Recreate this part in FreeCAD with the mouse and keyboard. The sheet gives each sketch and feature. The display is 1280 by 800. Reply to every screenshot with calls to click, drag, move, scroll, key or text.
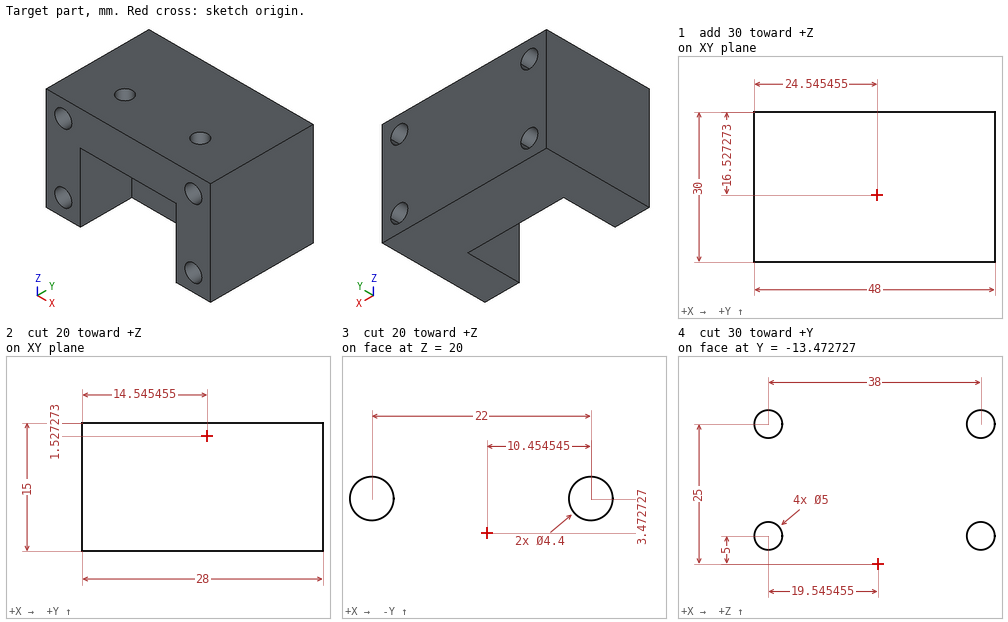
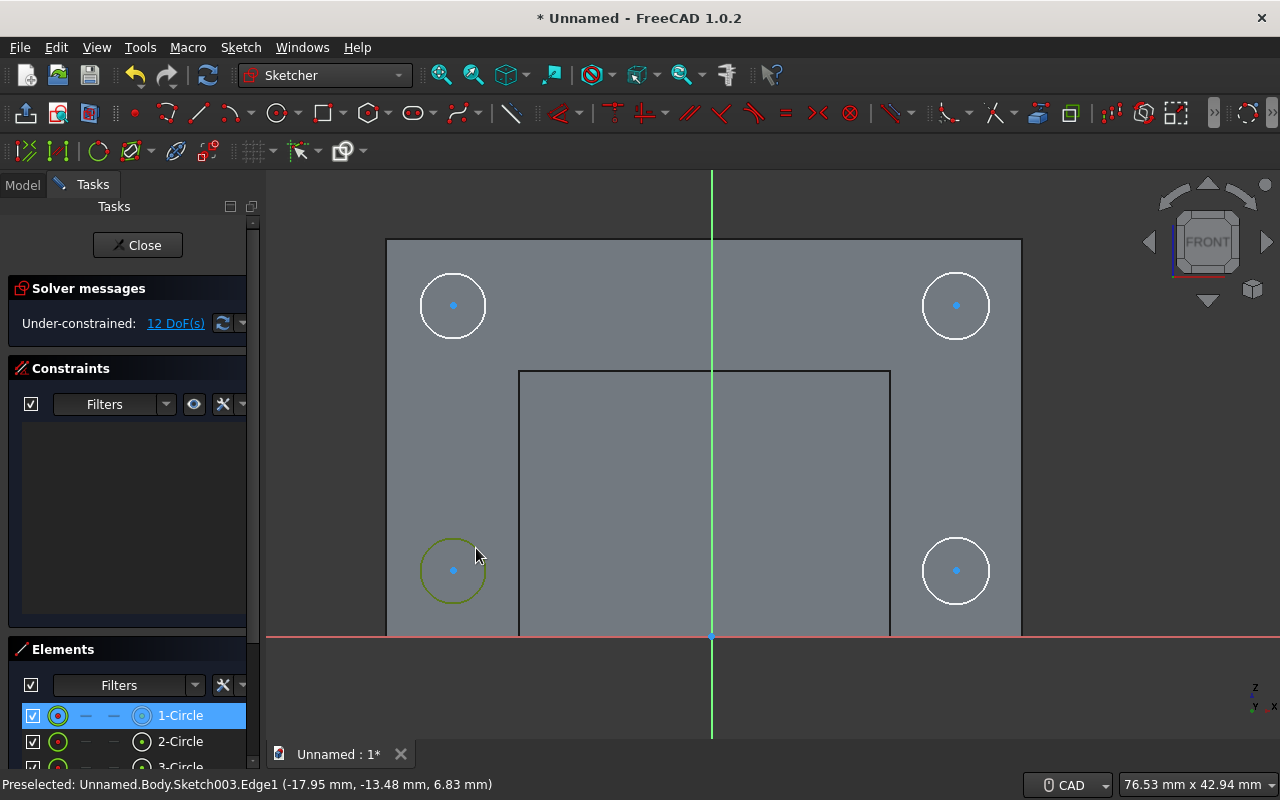
click(476, 283)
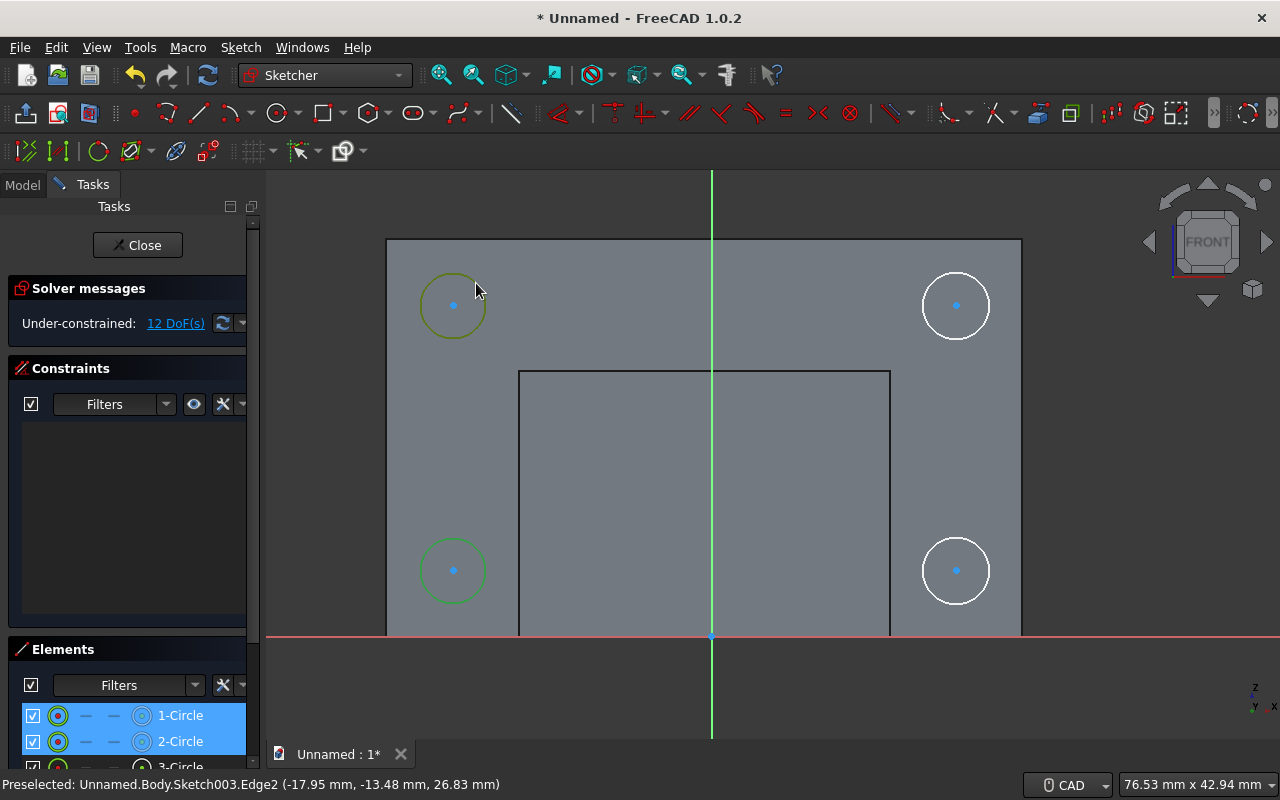
click(979, 282)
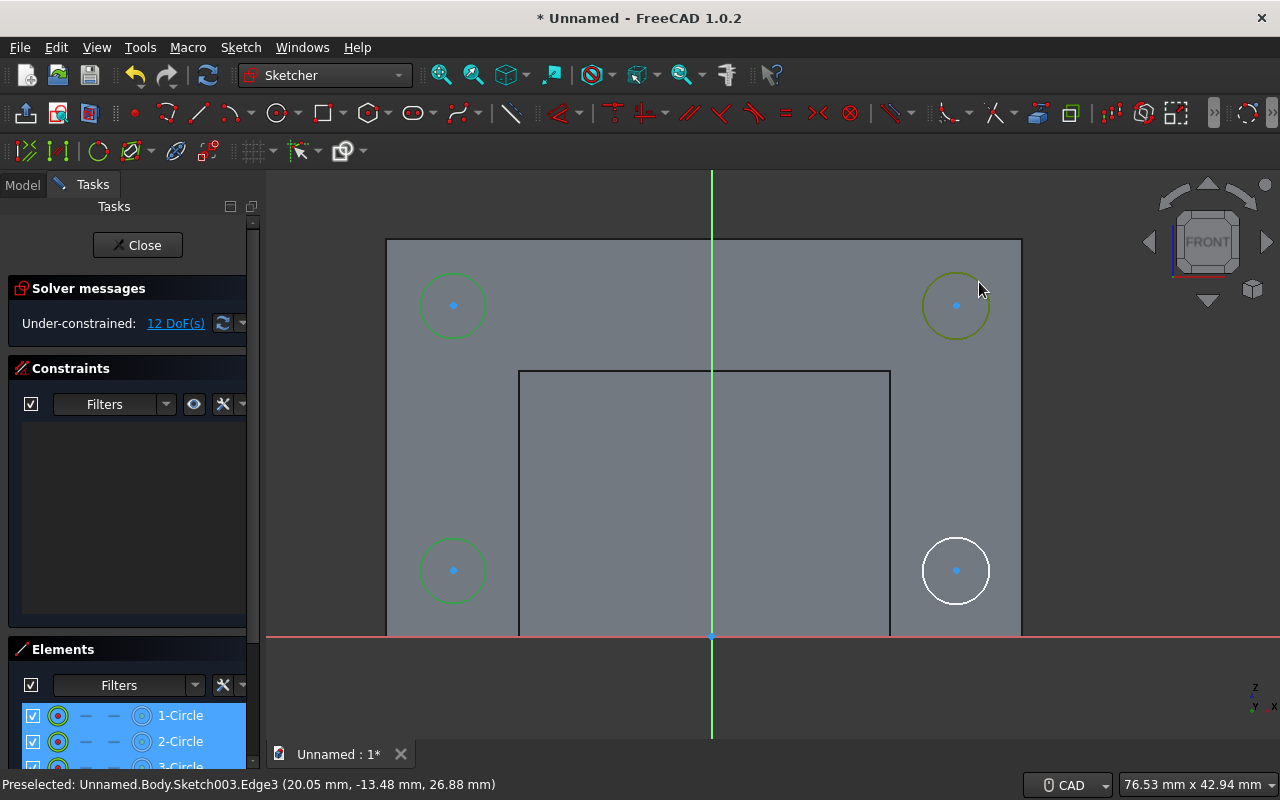
click(979, 547)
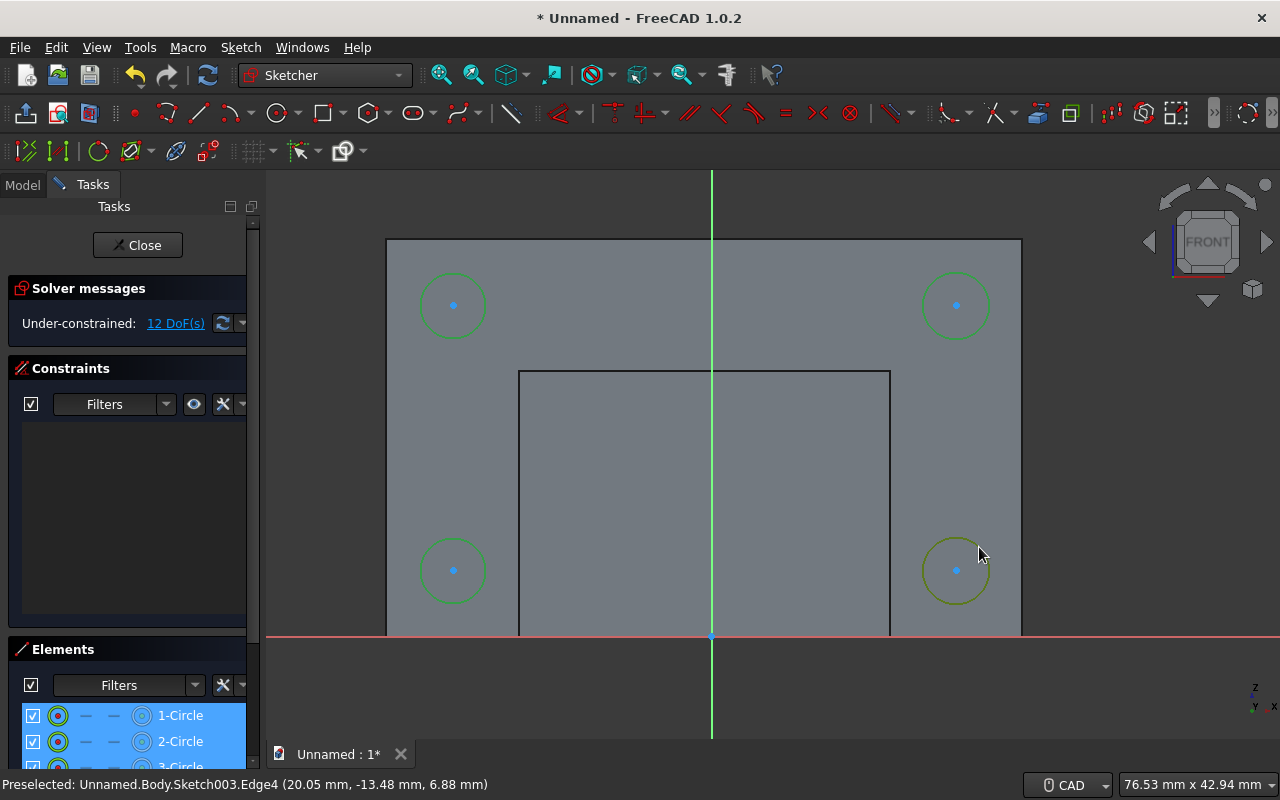
click(786, 114)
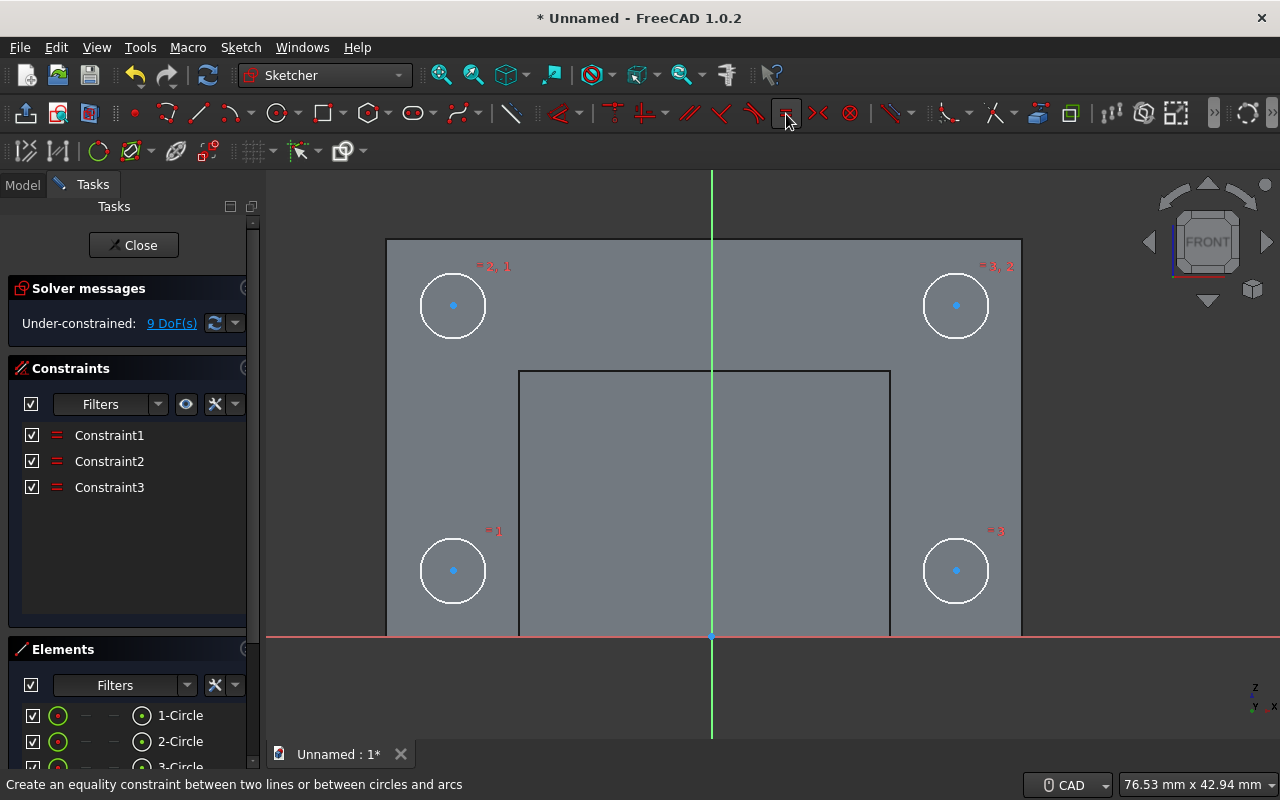
click(453, 571)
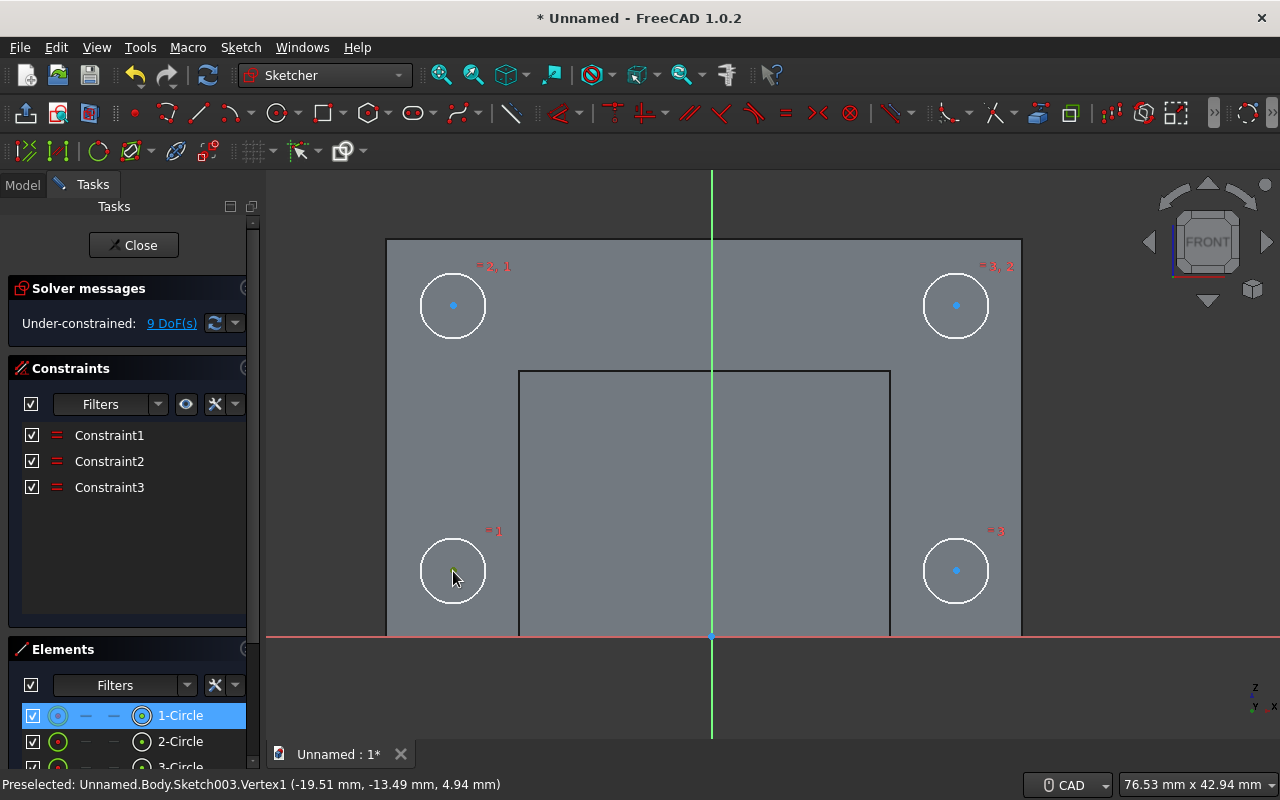
click(453, 306)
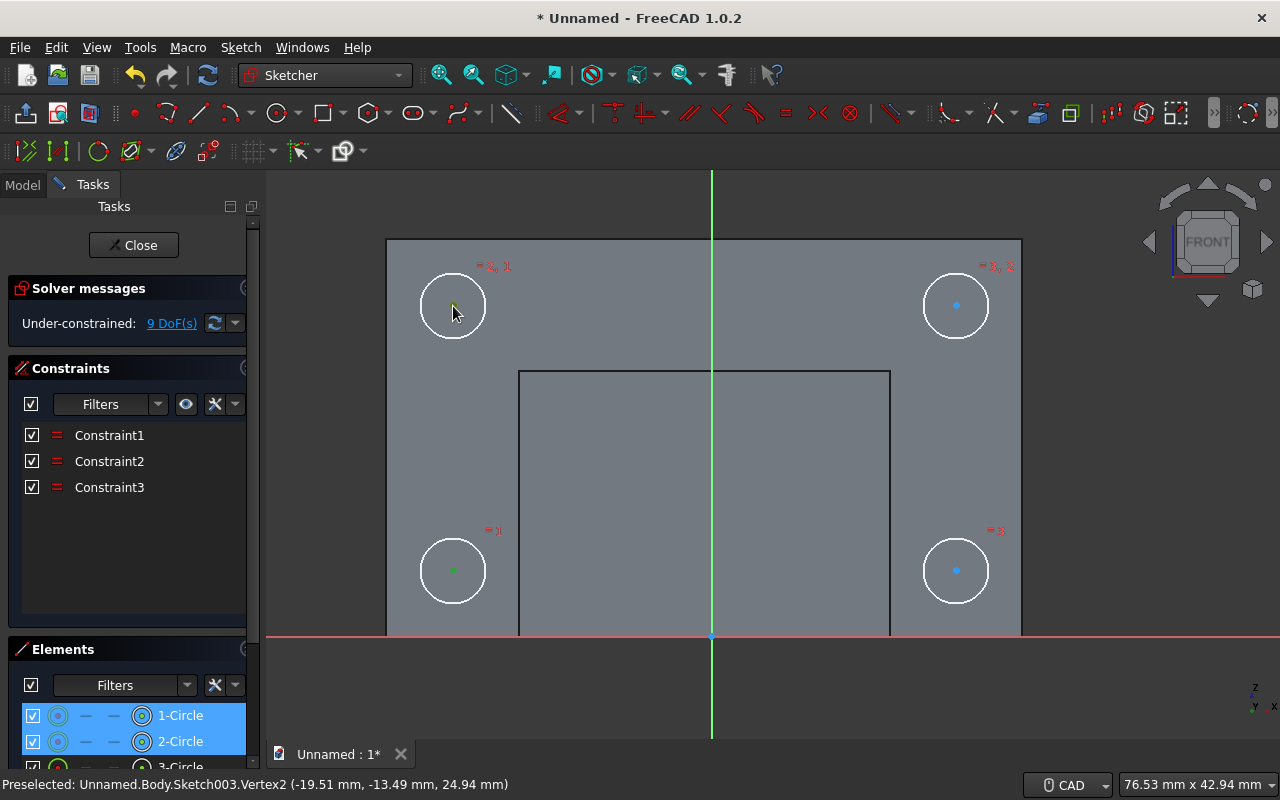
key(v)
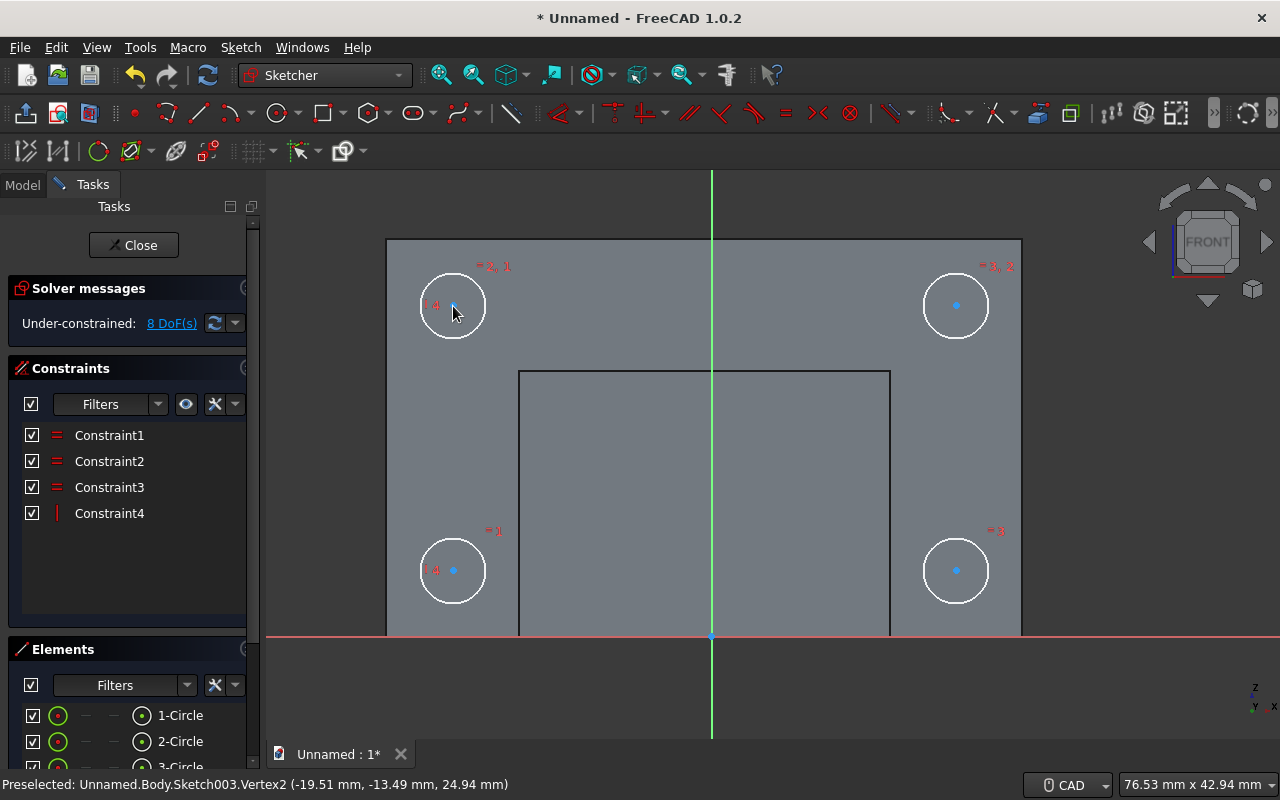
click(453, 306)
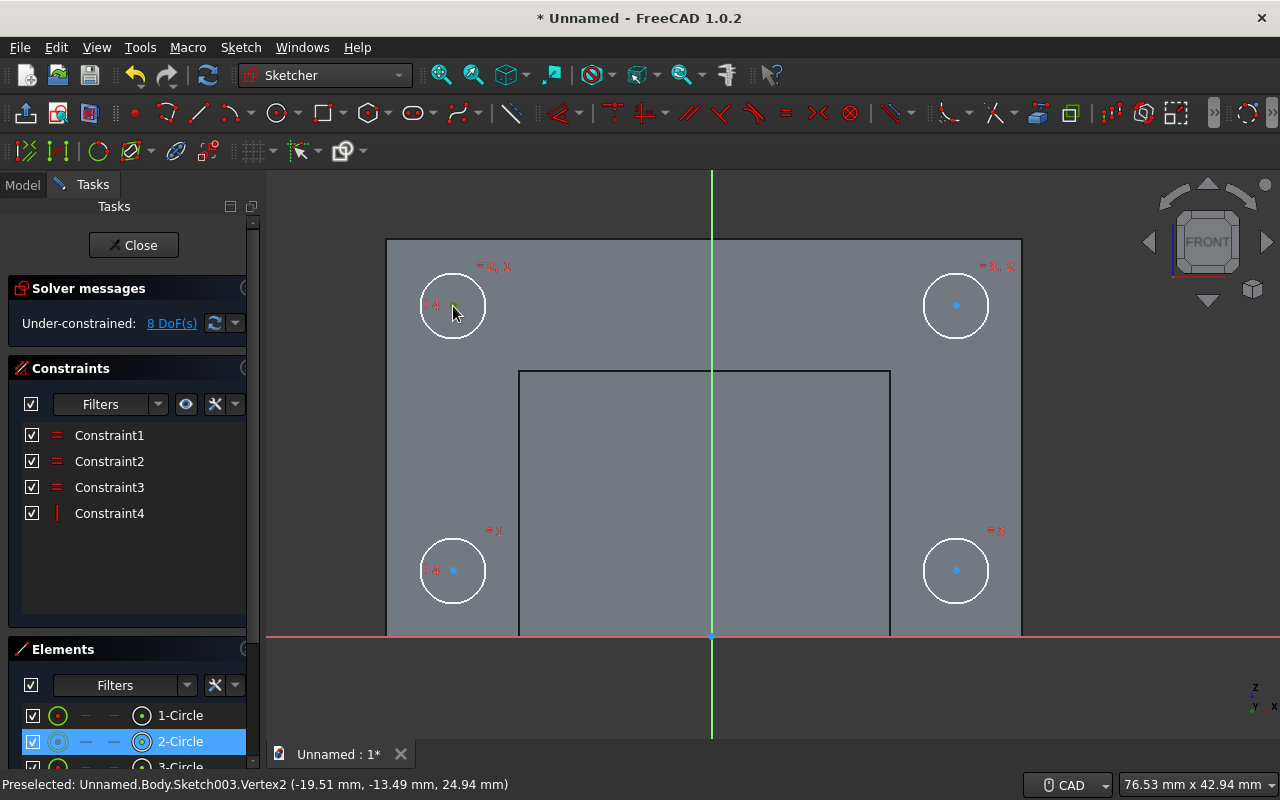
click(956, 306)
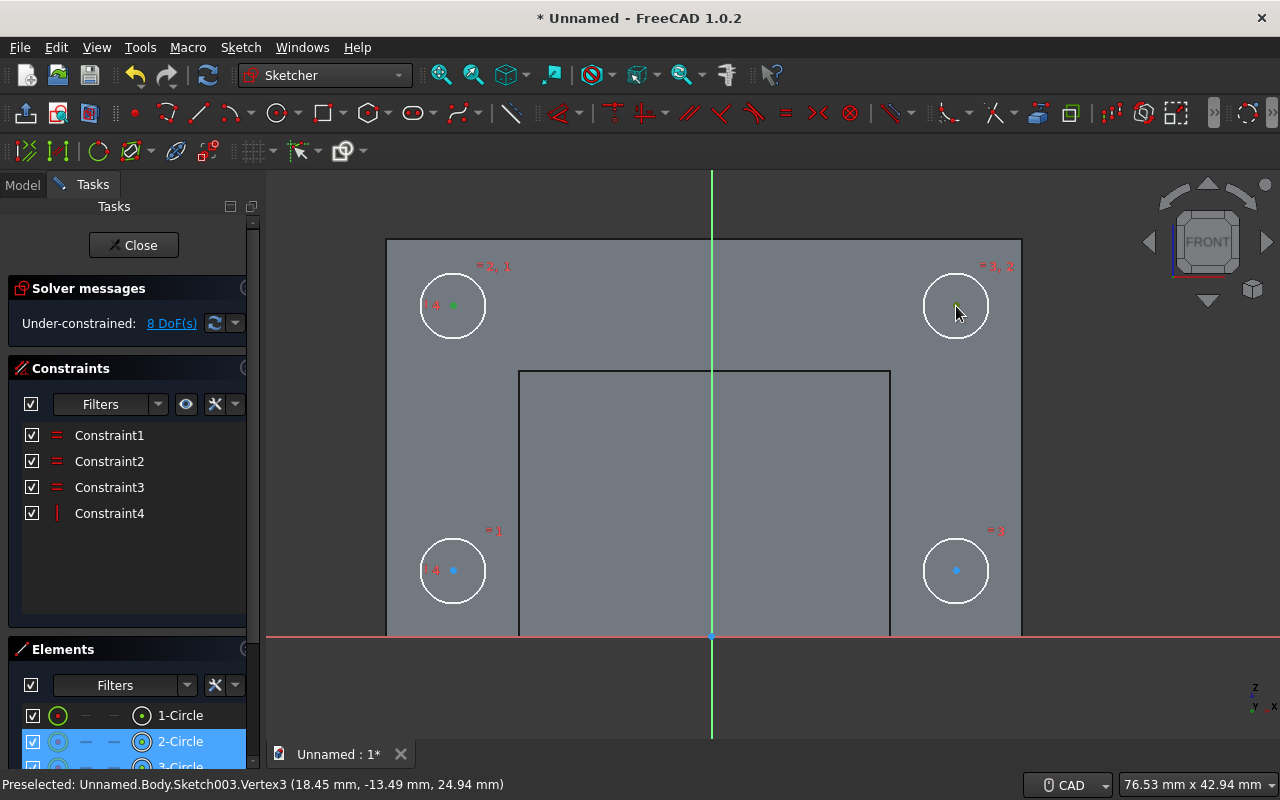
key(h)